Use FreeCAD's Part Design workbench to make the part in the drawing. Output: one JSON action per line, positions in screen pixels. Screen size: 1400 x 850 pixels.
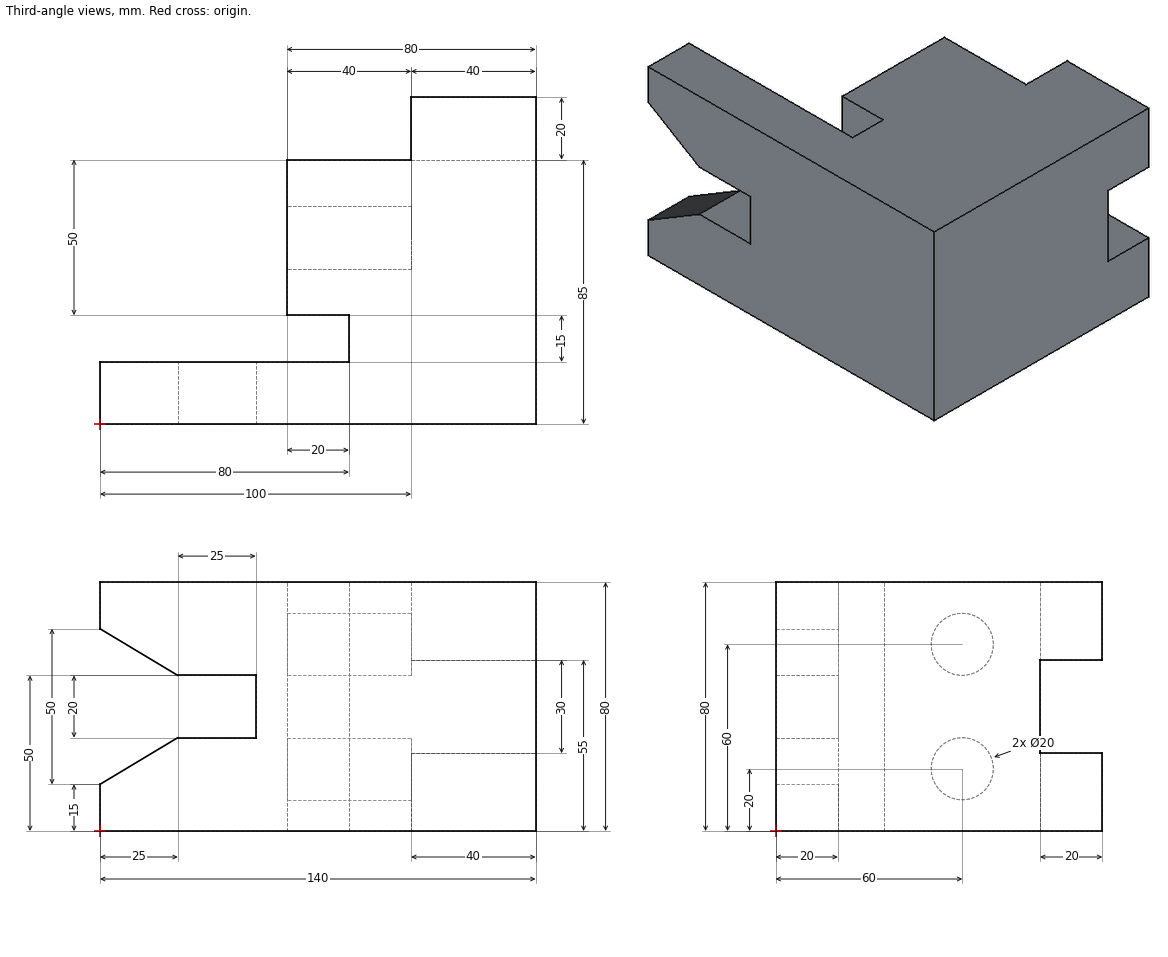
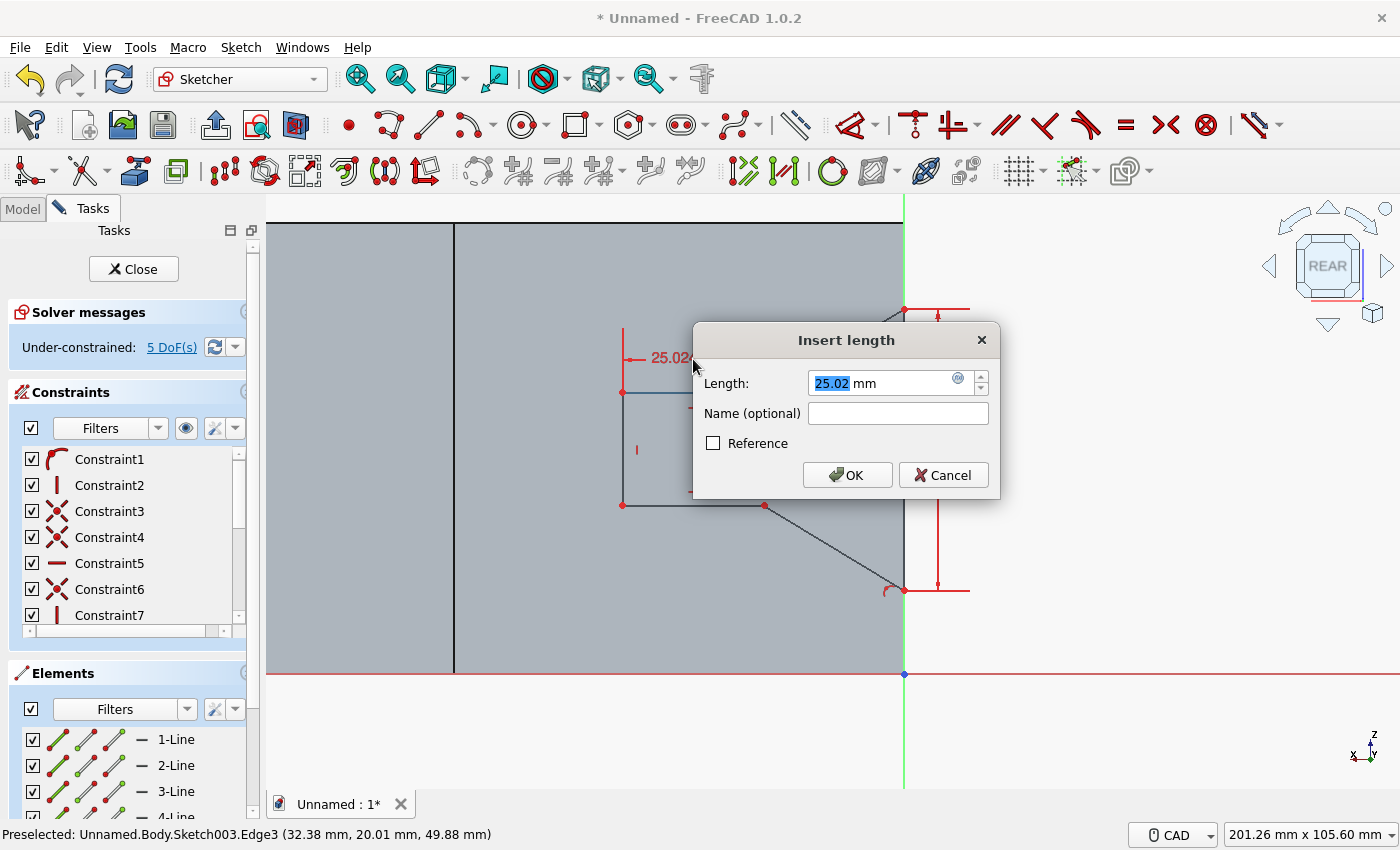
{"action": "type", "text": "25"}
{"action": "key", "text": "Return"}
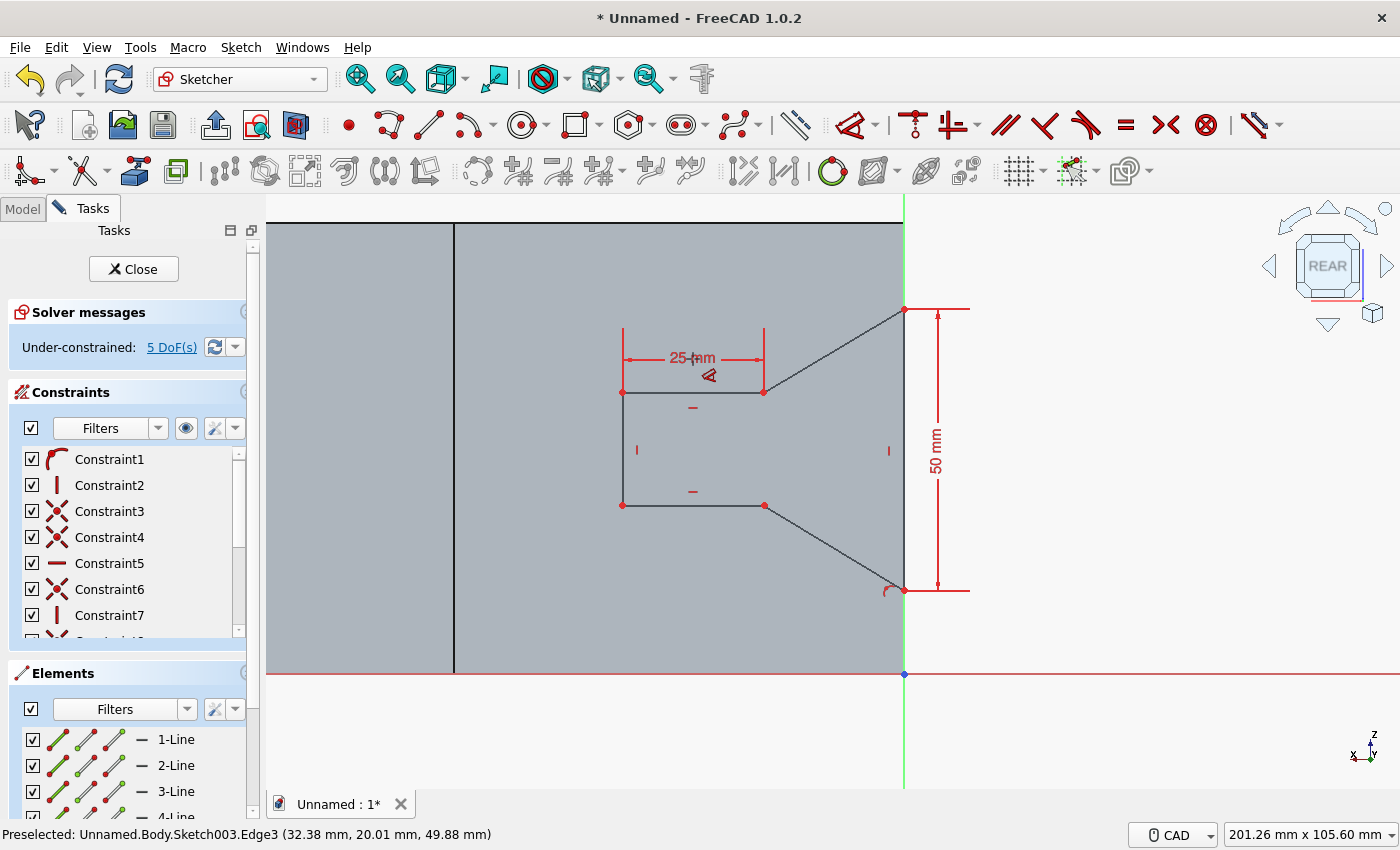
{"action": "left_click", "coordinate": [623, 427]}
{"action": "left_click", "coordinate": [589, 449]}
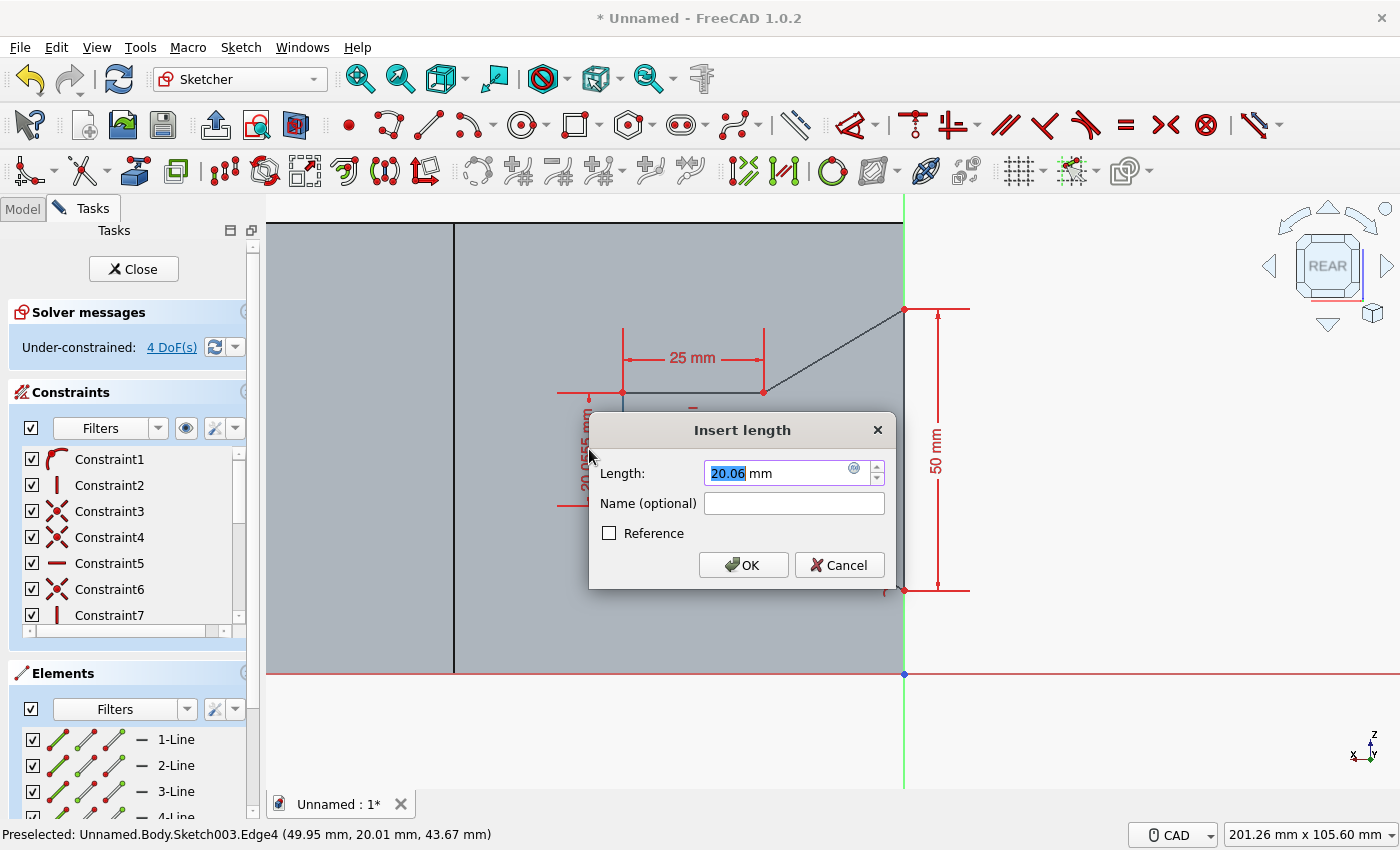
{"action": "type", "text": "20"}
{"action": "key", "text": "Return"}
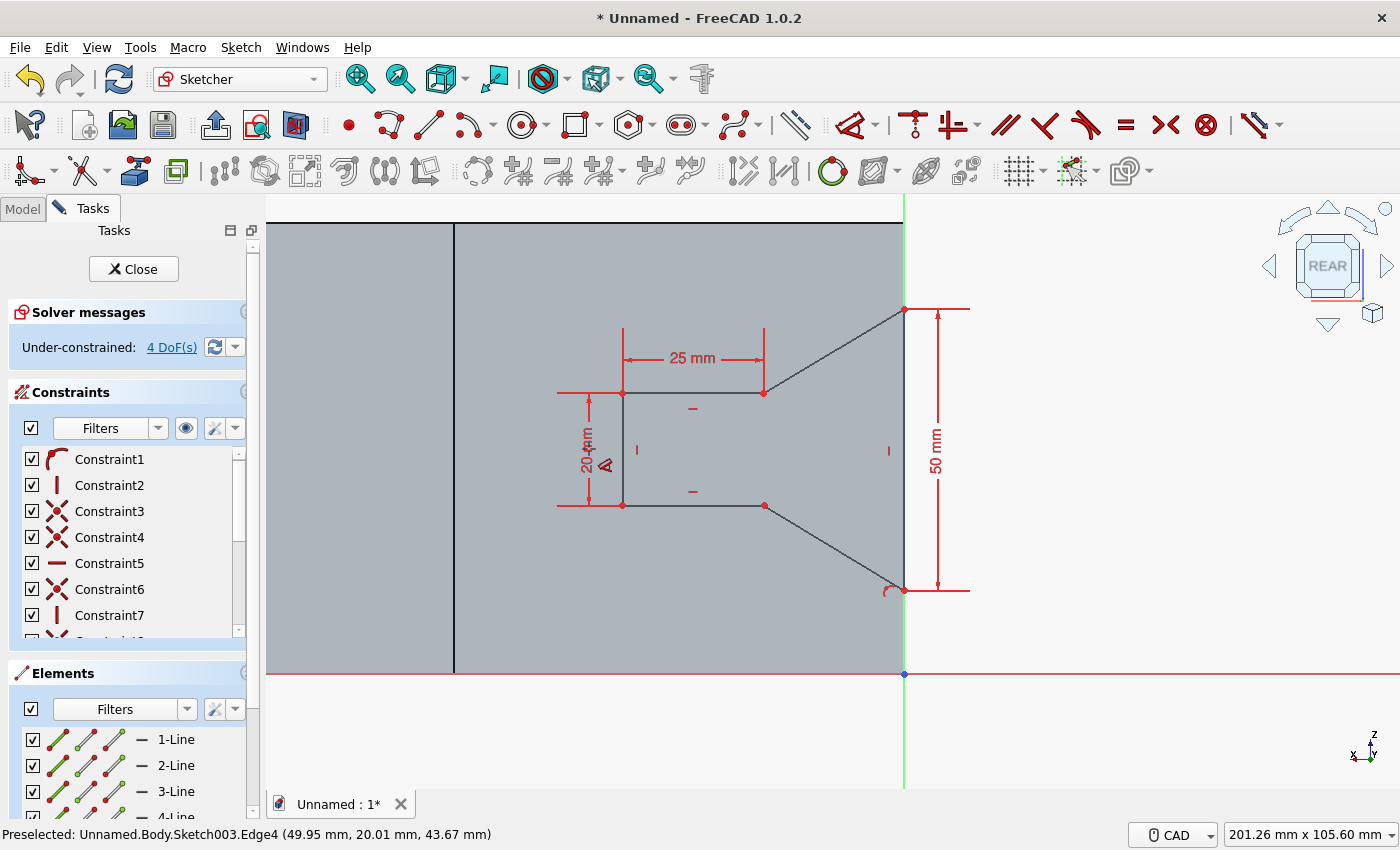
{"action": "left_click", "coordinate": [665, 506]}
{"action": "left_click", "coordinate": [693, 540]}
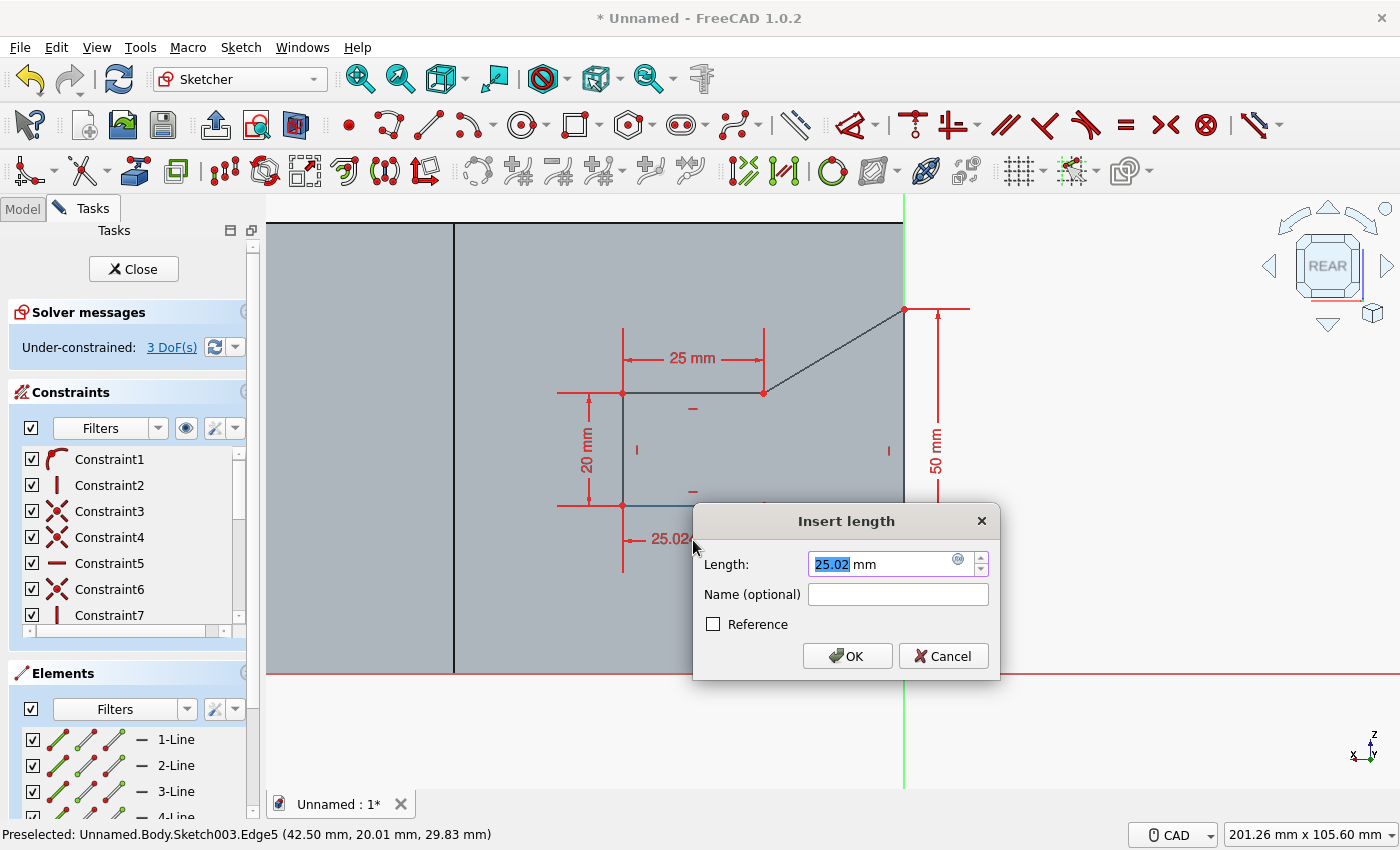
{"action": "type", "text": "25"}
{"action": "key", "text": "Return"}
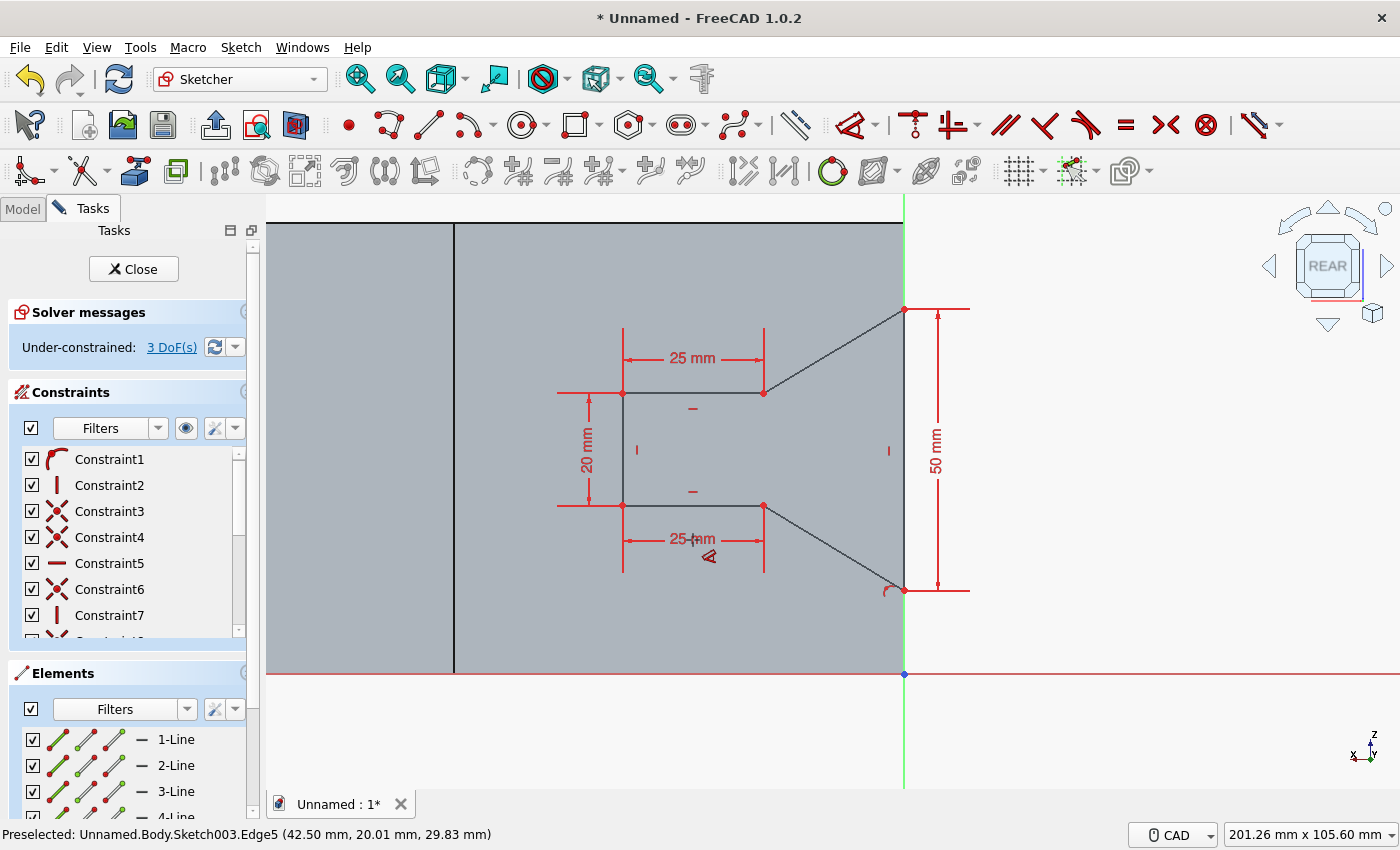
{"action": "left_click", "coordinate": [904, 591]}
{"action": "left_click", "coordinate": [938, 633]}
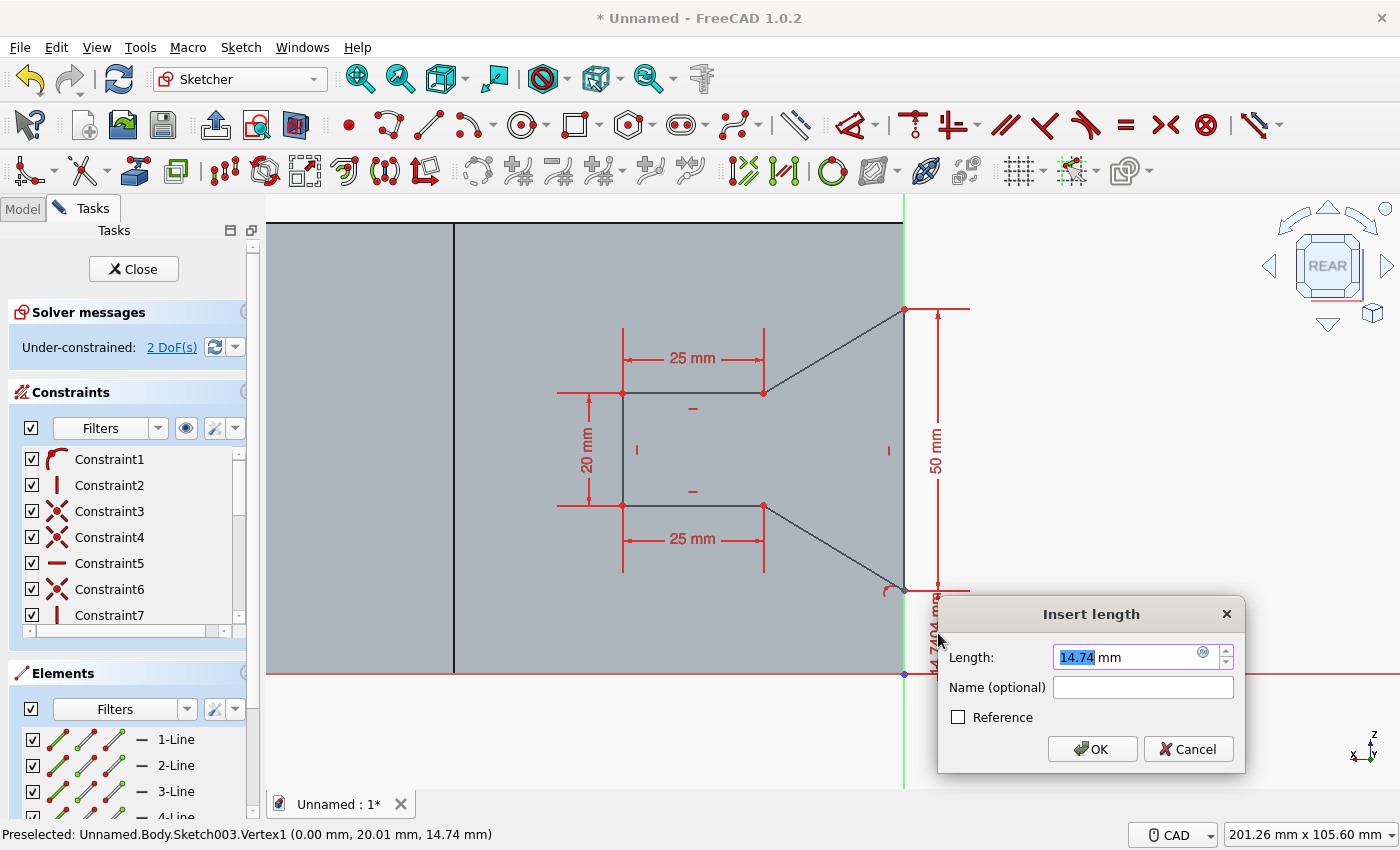
{"action": "type", "text": "15"}
{"action": "key", "text": "Return"}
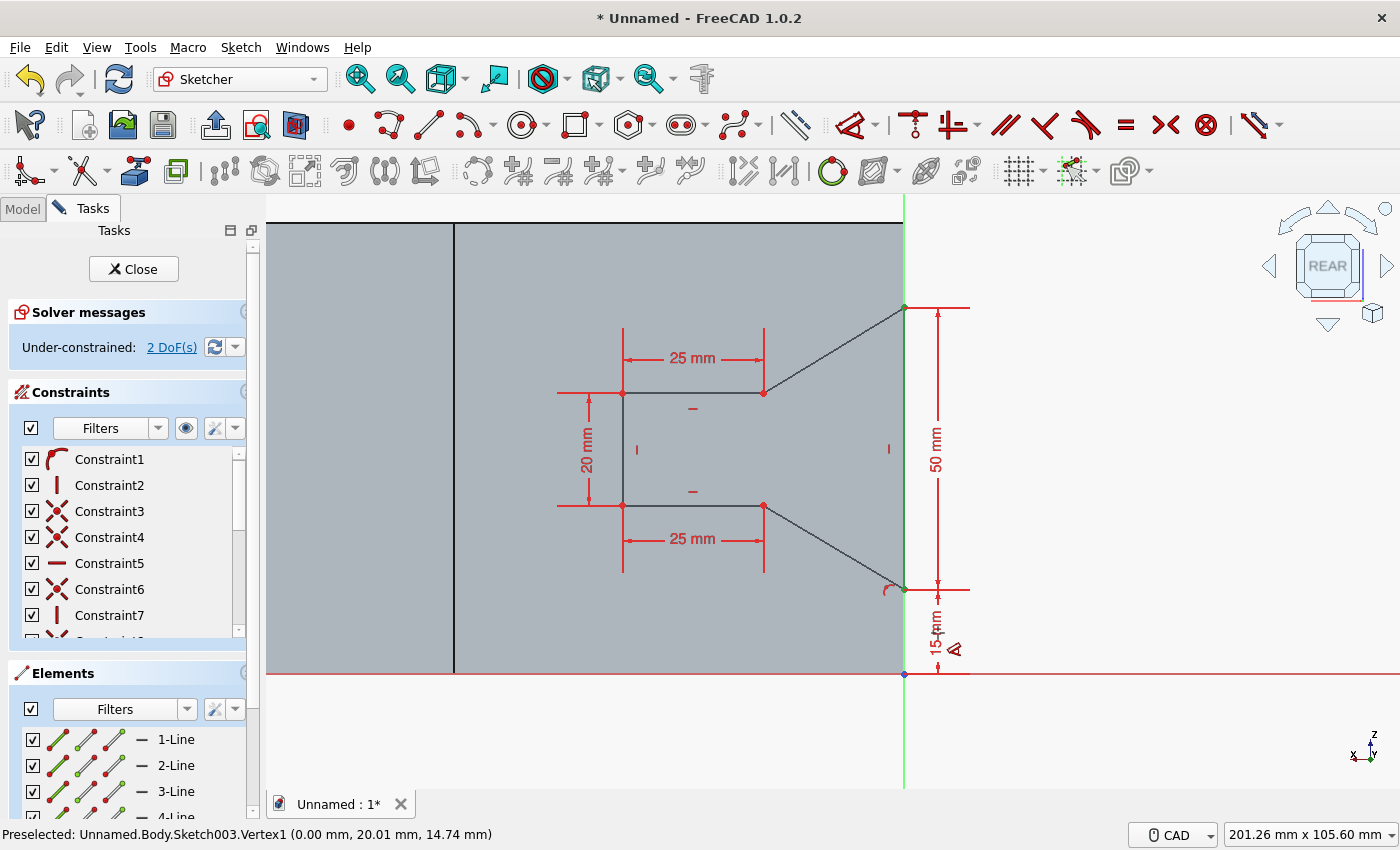
{"action": "left_click", "coordinate": [764, 393]}
{"action": "left_click", "coordinate": [834, 708]}